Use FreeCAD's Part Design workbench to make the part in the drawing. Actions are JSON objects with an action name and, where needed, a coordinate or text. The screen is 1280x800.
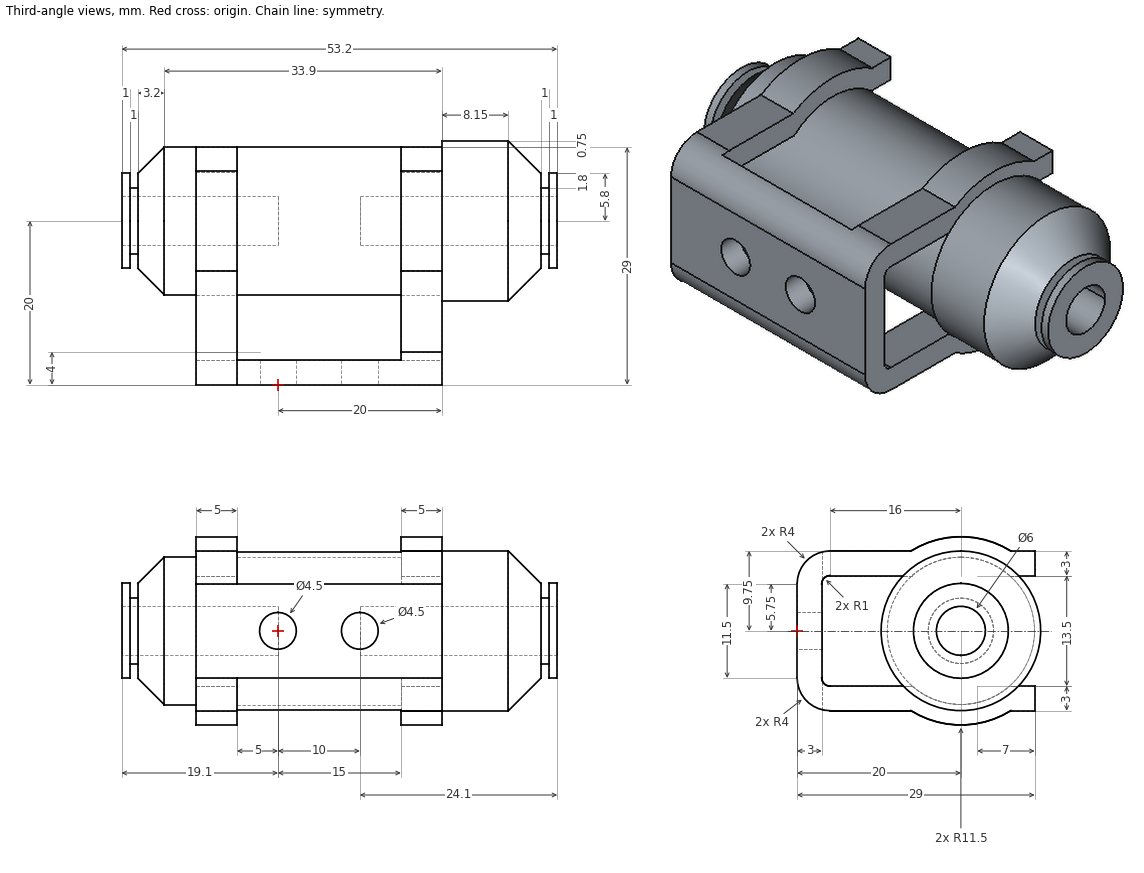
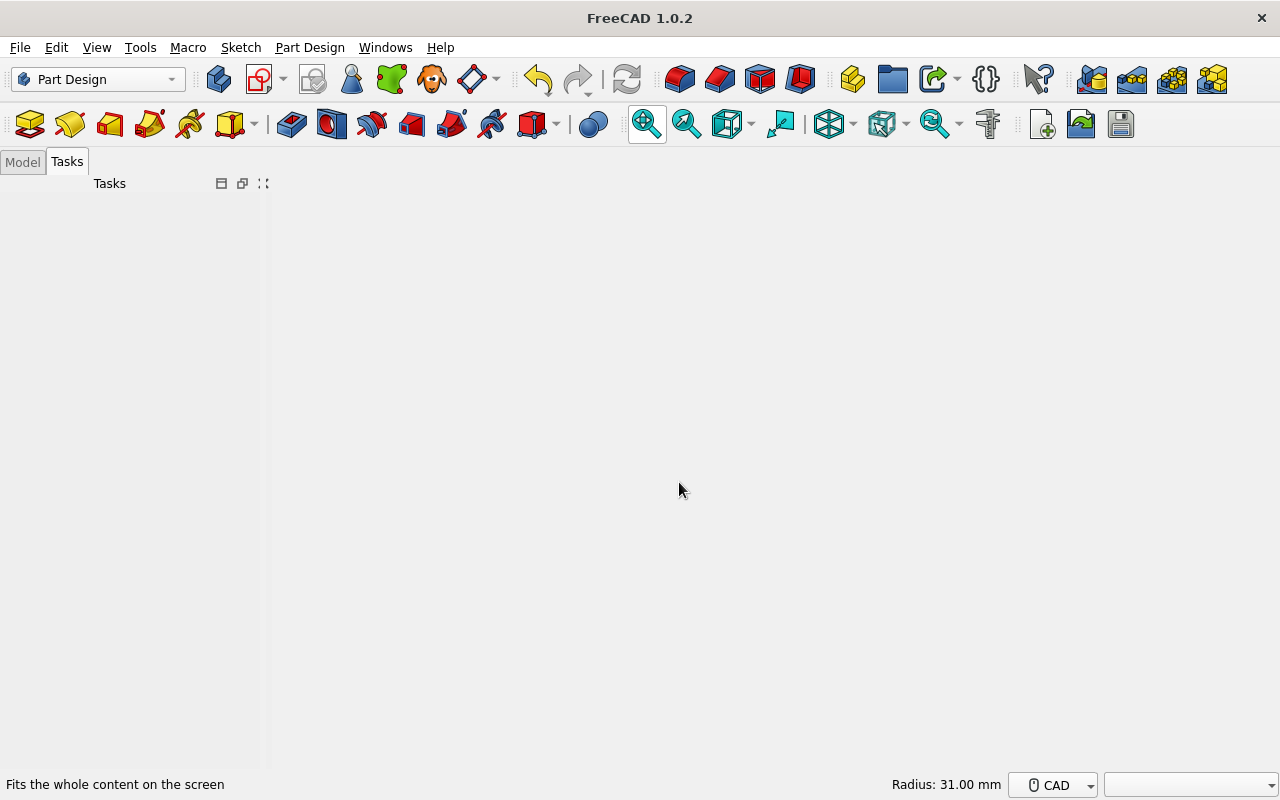
{"action": "left_click", "coordinate": [1042, 124]}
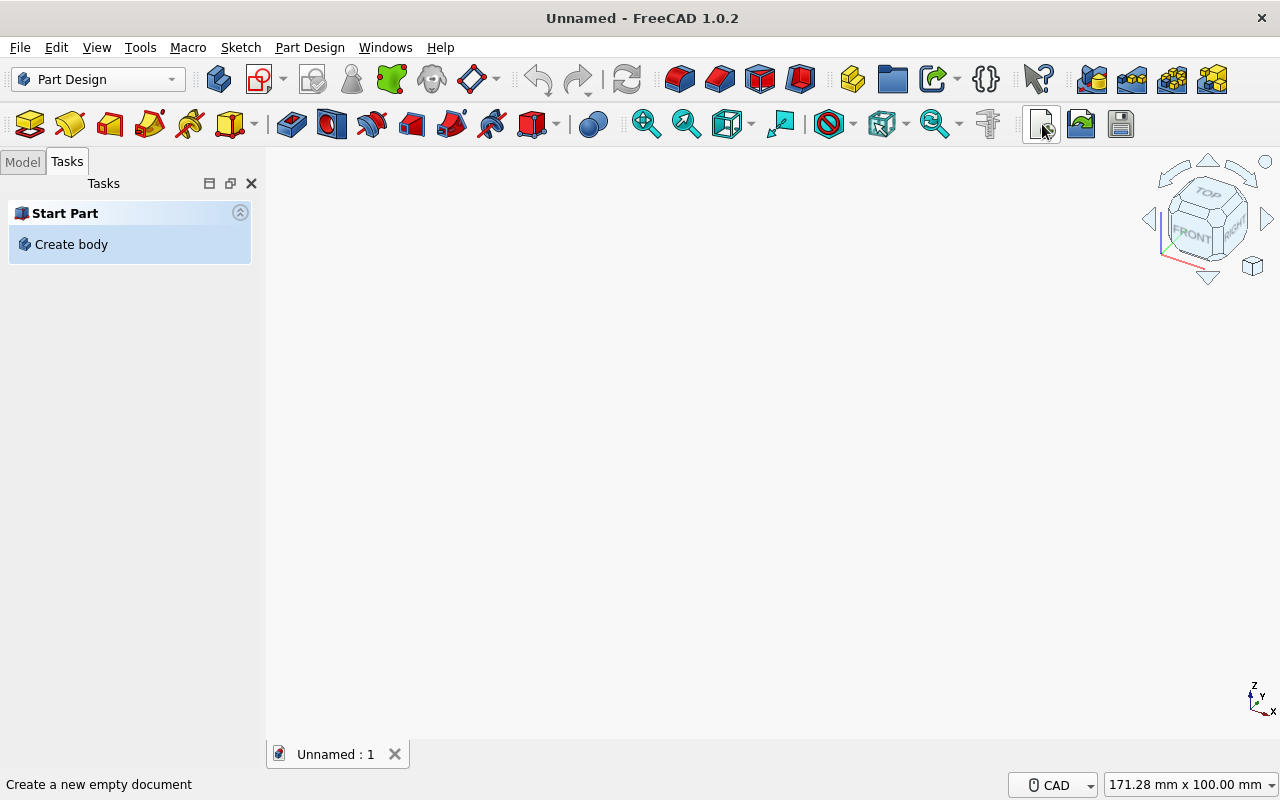
{"action": "left_click", "coordinate": [260, 80]}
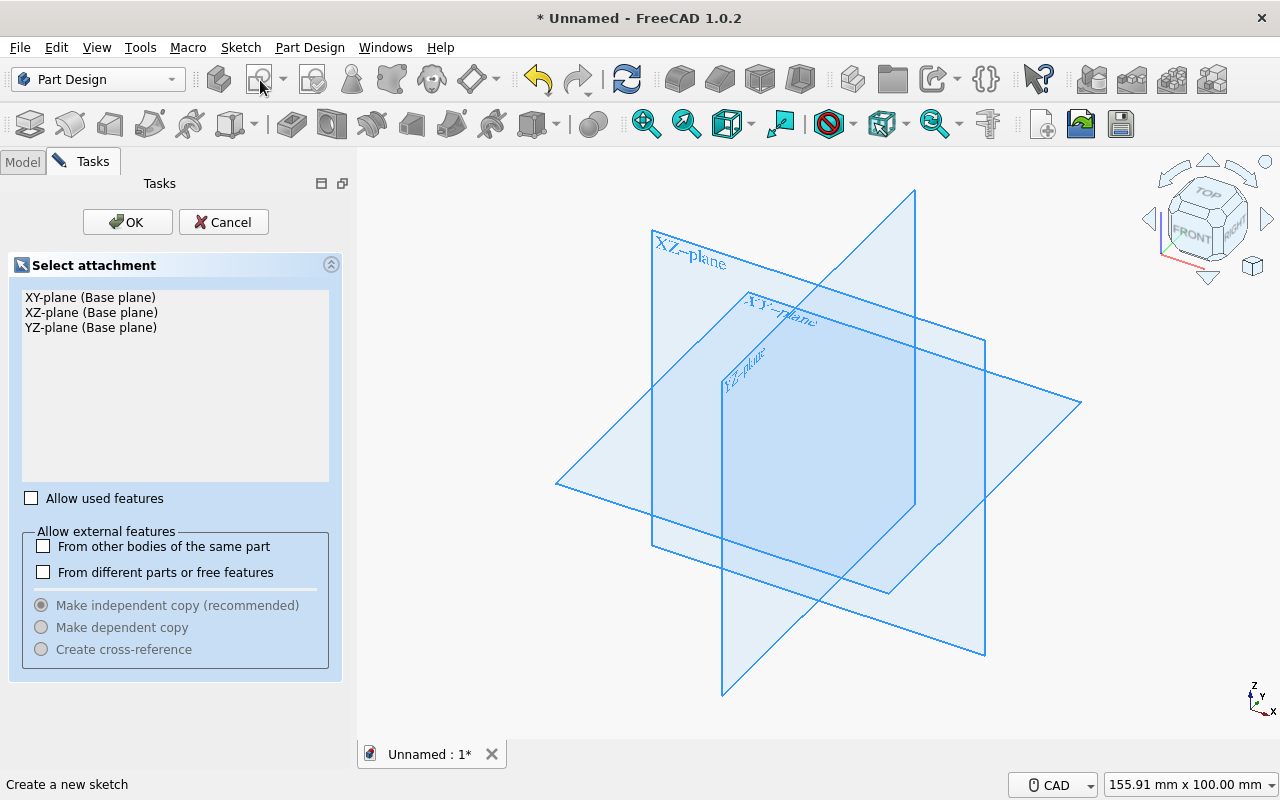
{"action": "left_click", "coordinate": [82, 298]}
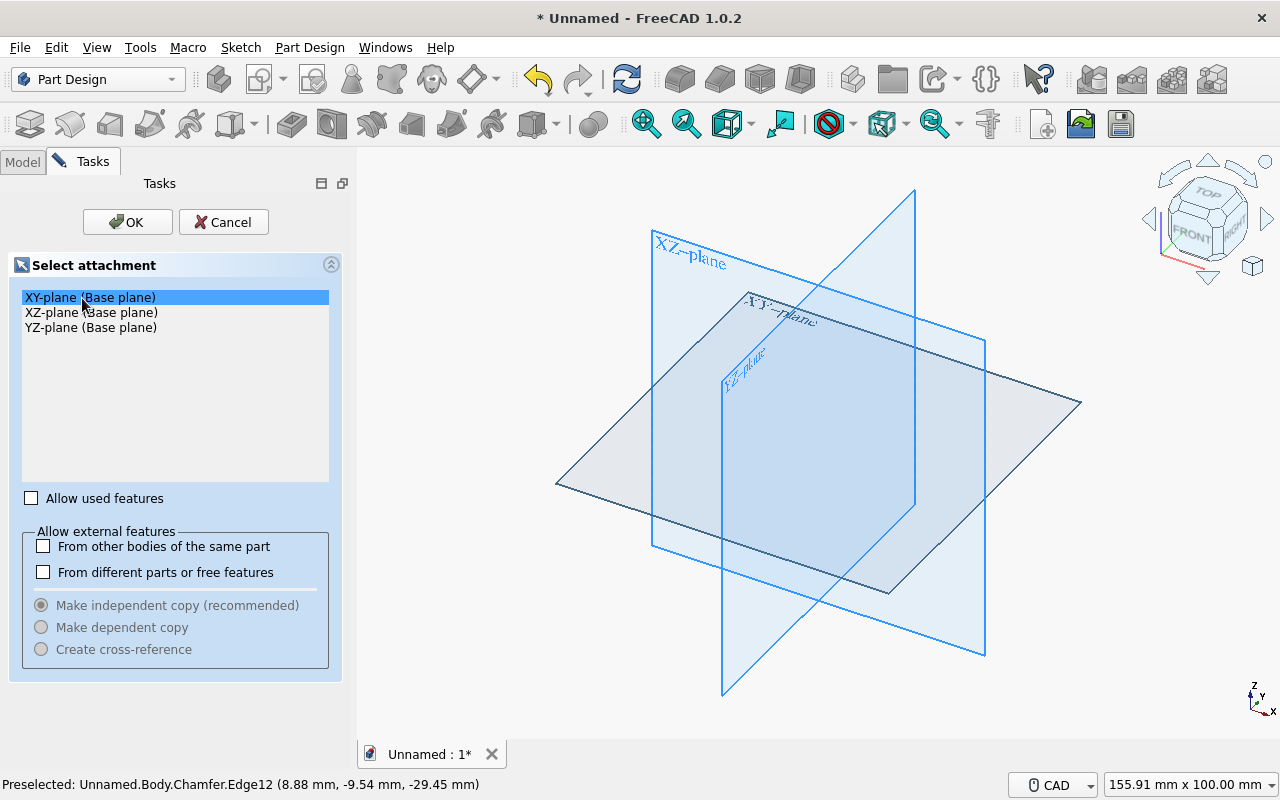
{"action": "left_click", "coordinate": [128, 222]}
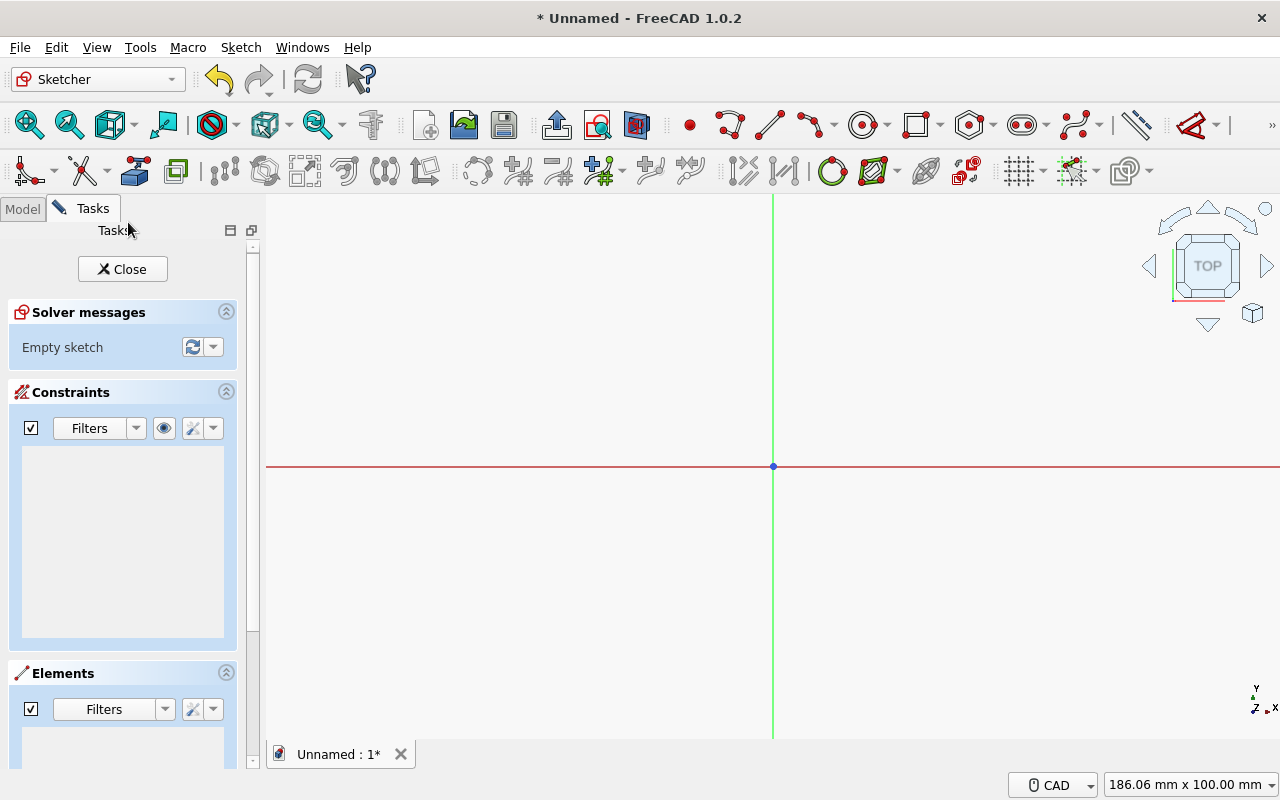
{"action": "scroll", "coordinate": [860, 222], "scroll_direction": "up", "scroll_amount": 2}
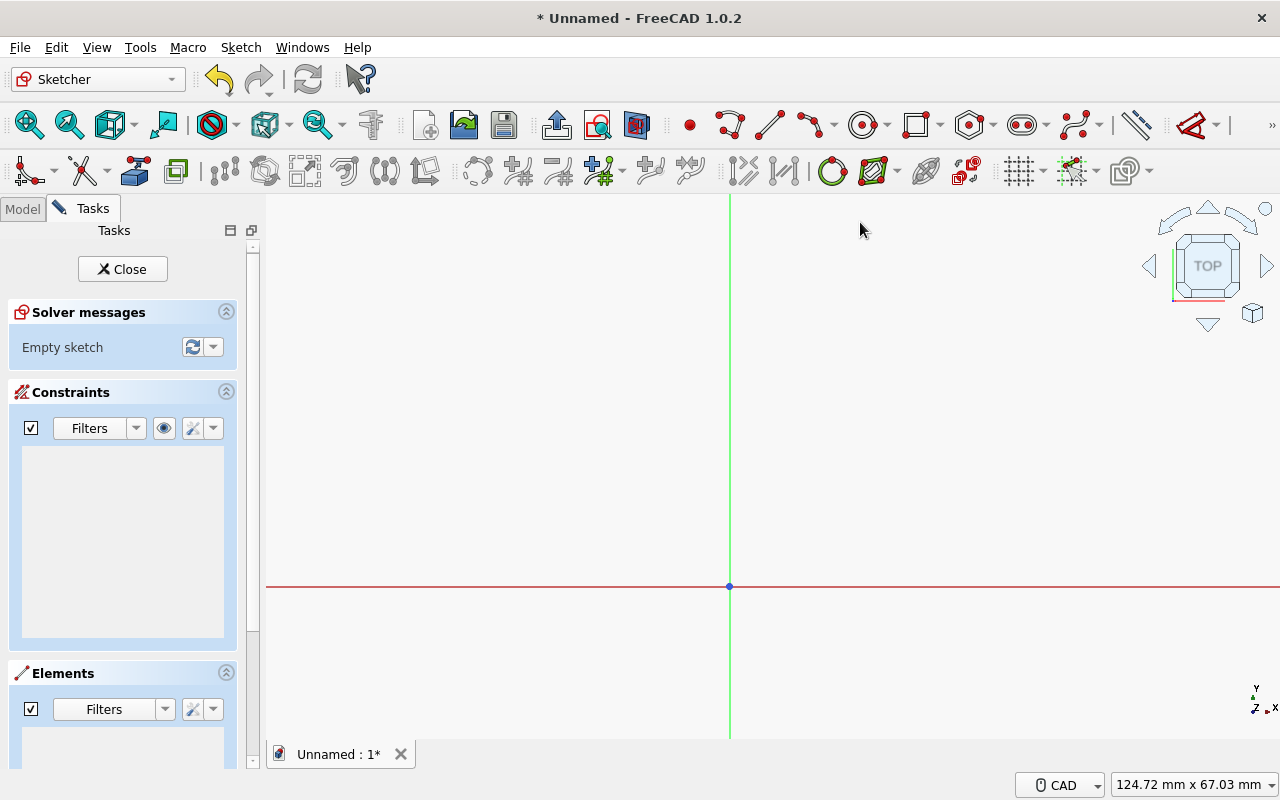
{"action": "left_click", "coordinate": [730, 126]}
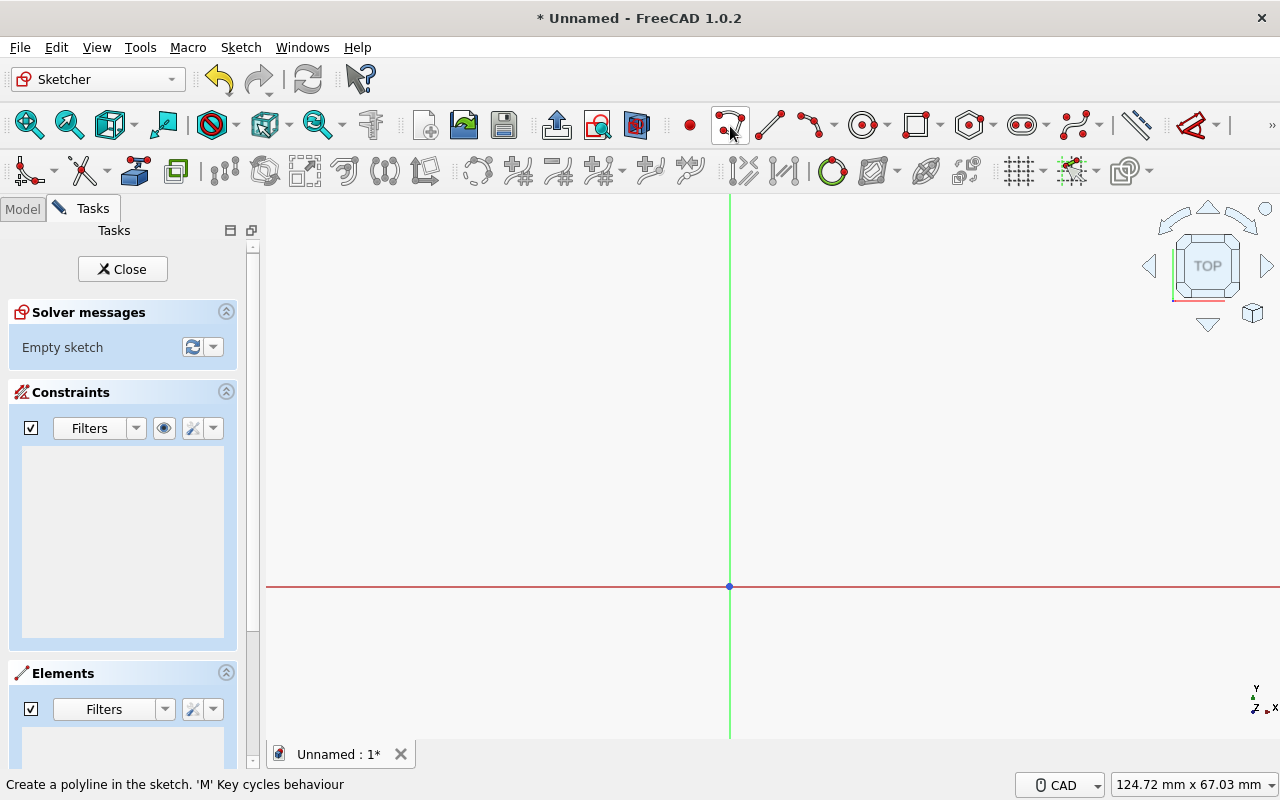
{"action": "left_click", "coordinate": [575, 424]}
{"action": "left_click", "coordinate": [1007, 424]}
{"action": "left_click", "coordinate": [1007, 377]}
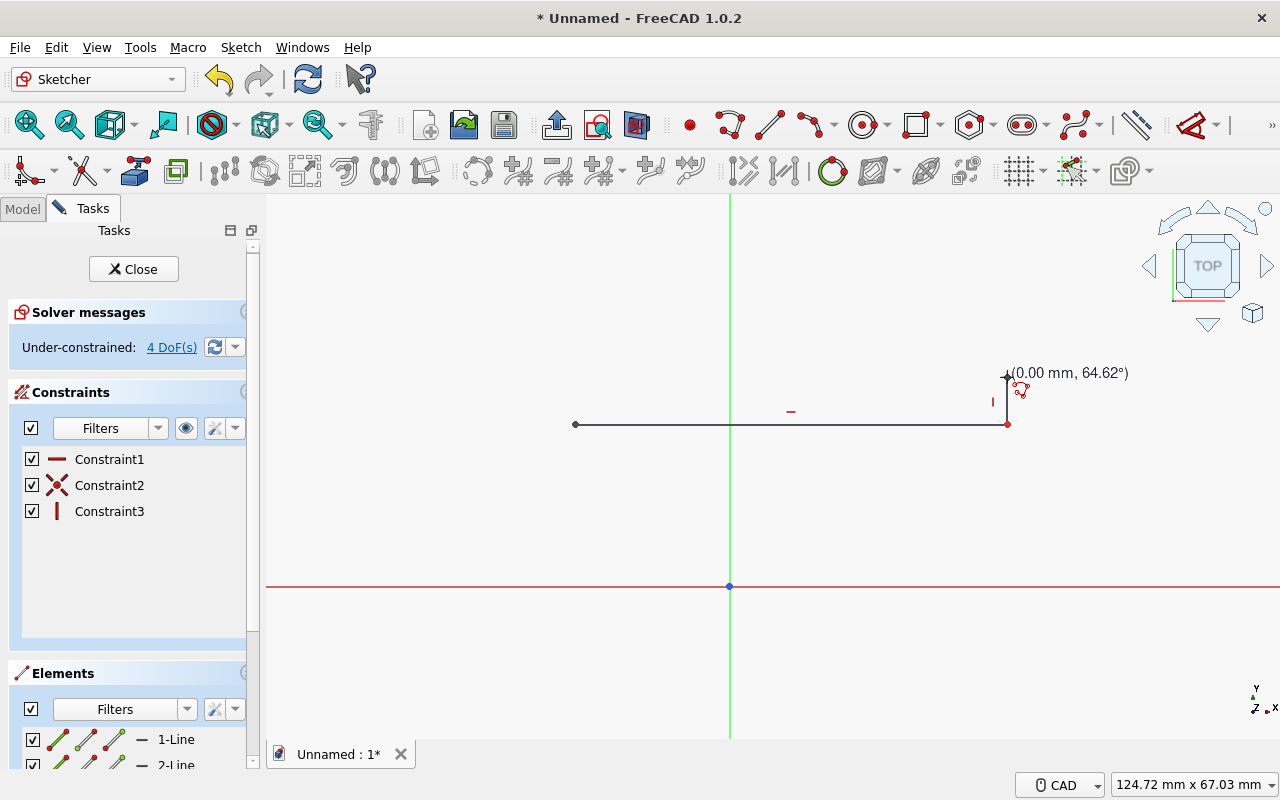
{"action": "scroll", "coordinate": [999, 377], "scroll_direction": "up", "scroll_amount": 4}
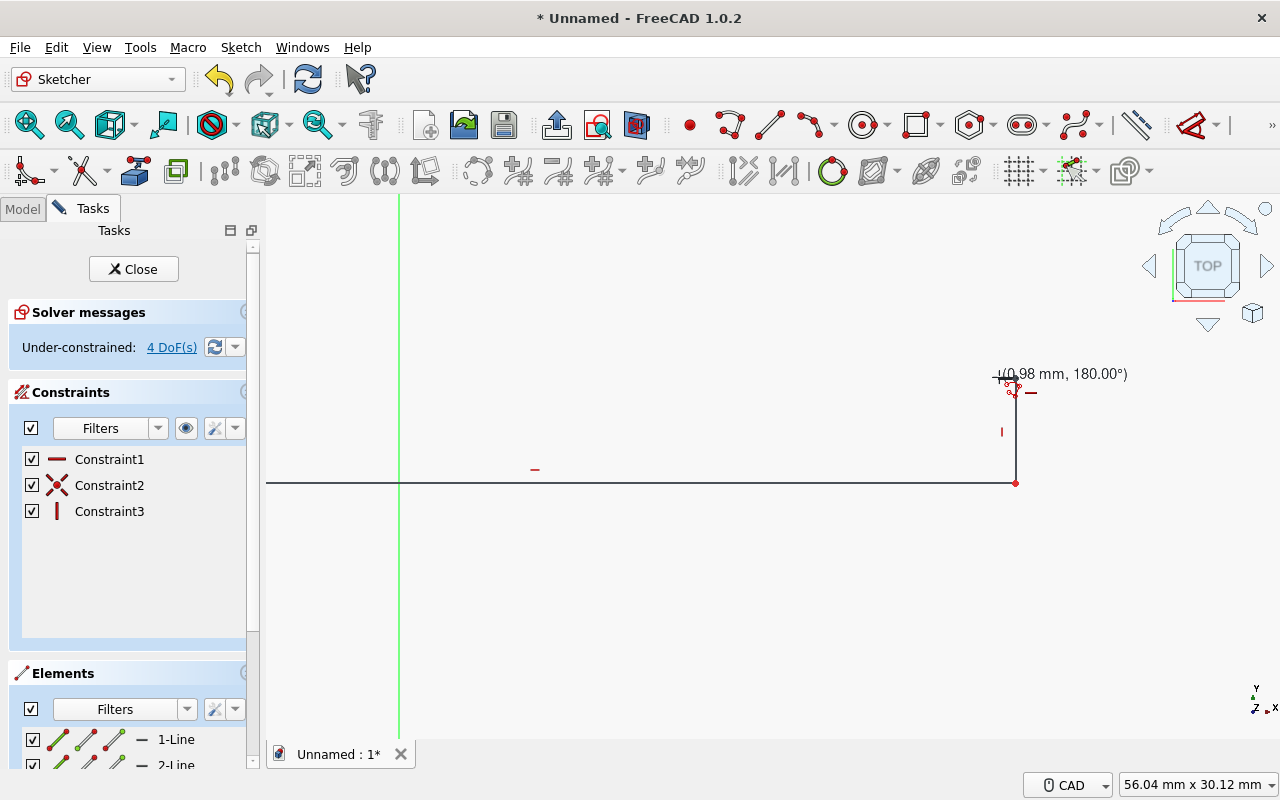
{"action": "left_click", "coordinate": [998, 377]}
{"action": "left_click", "coordinate": [998, 409]}
{"action": "left_click", "coordinate": [980, 409]}
{"action": "left_click", "coordinate": [980, 376]}
{"action": "left_click", "coordinate": [909, 305]}
{"action": "left_click", "coordinate": [761, 305]}
{"action": "left_click", "coordinate": [761, 319]}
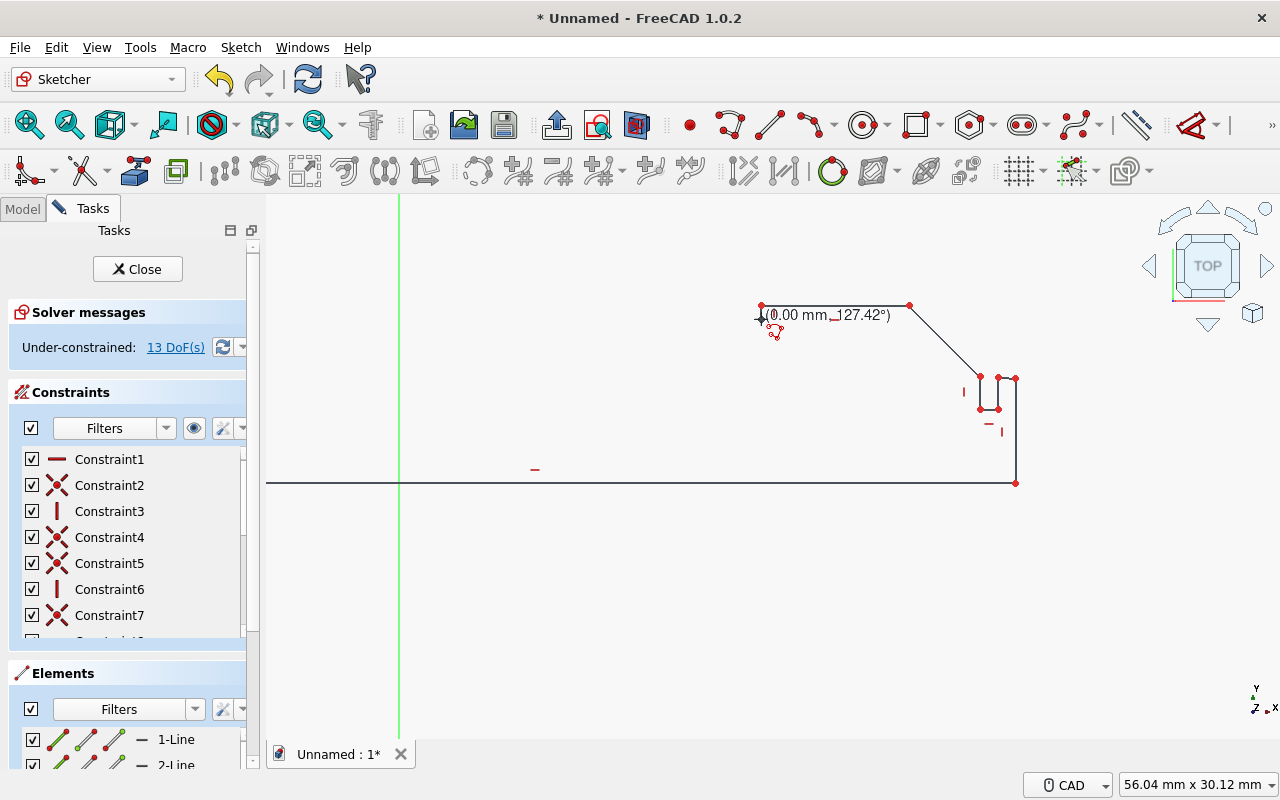
{"action": "scroll", "coordinate": [1000, 379], "scroll_direction": "down", "scroll_amount": 4}